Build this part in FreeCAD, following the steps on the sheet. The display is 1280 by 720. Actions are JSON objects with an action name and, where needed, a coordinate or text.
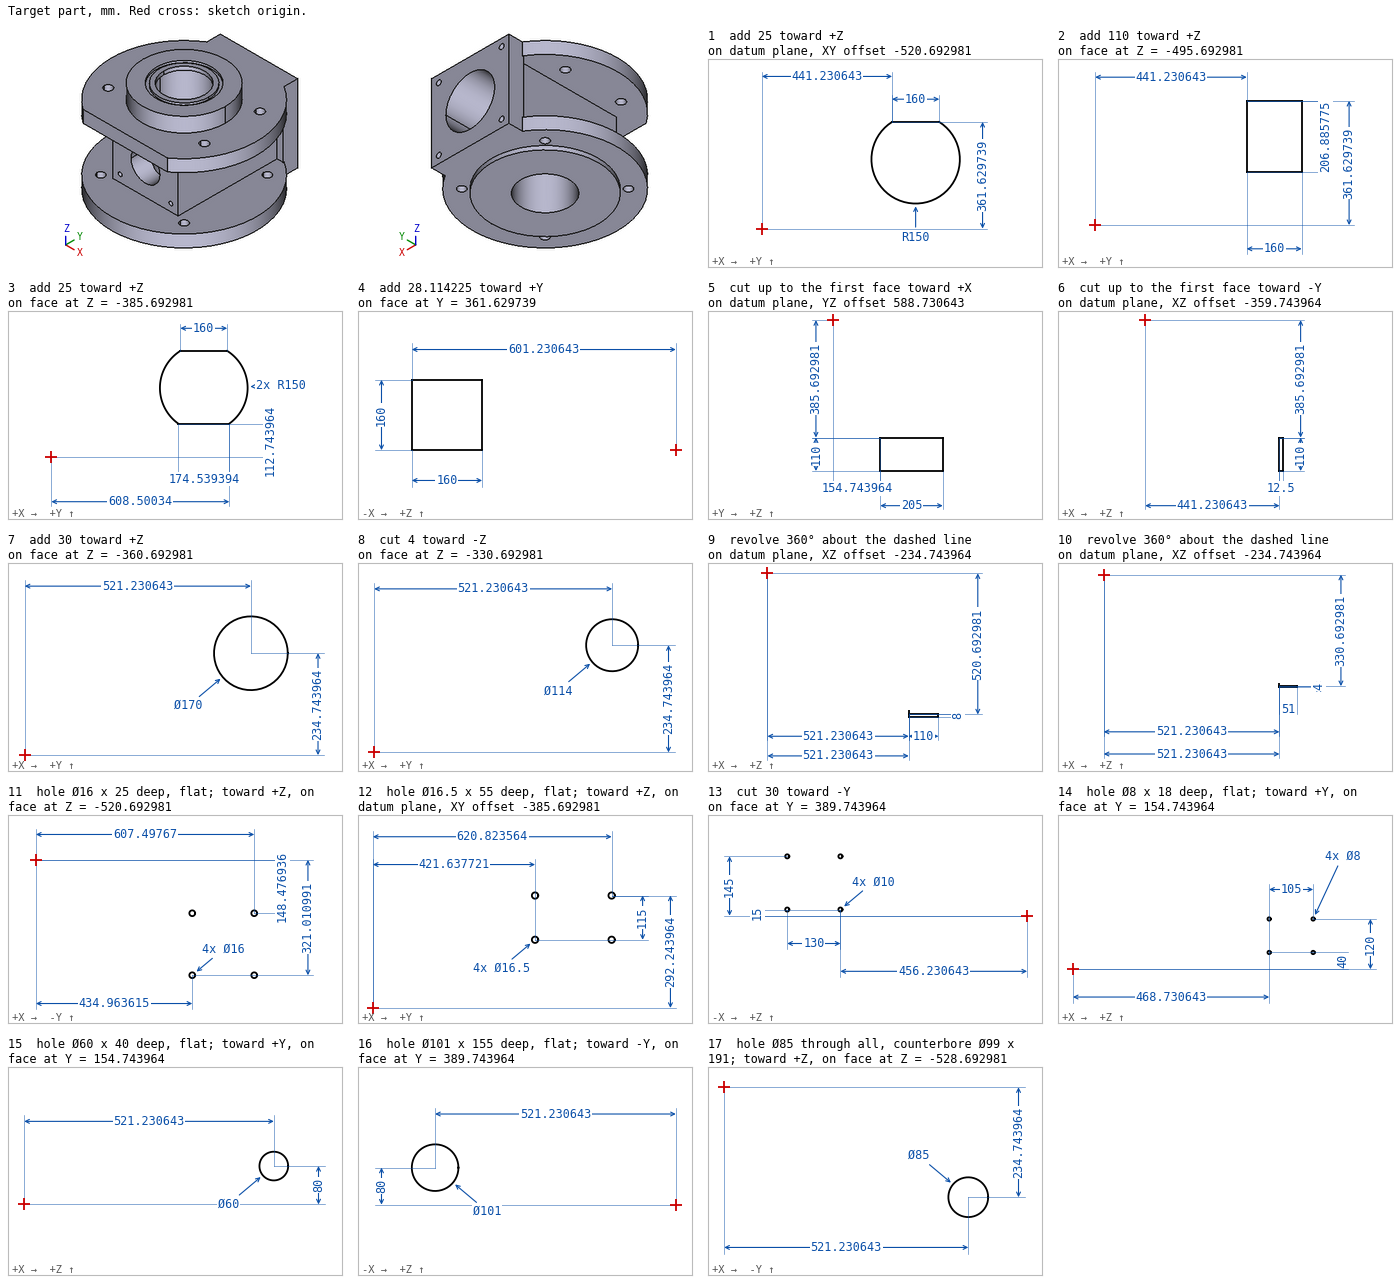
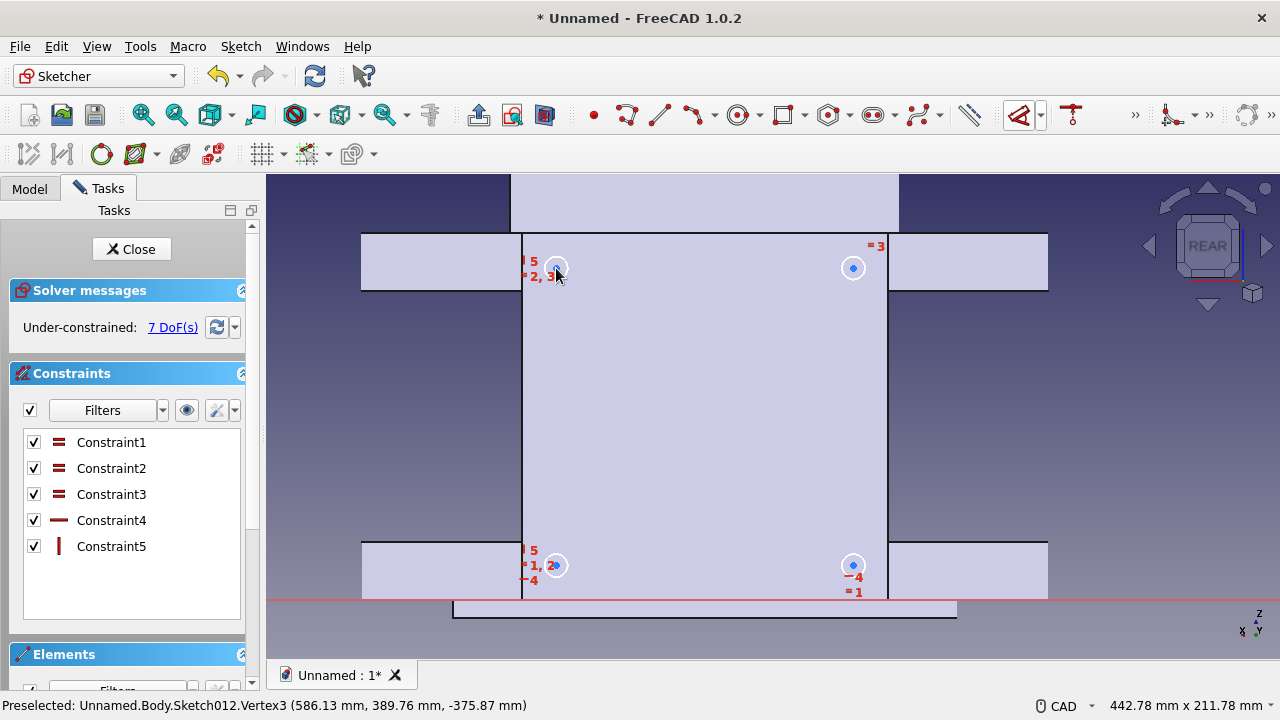
{"action": "left_click", "coordinate": [854, 566]}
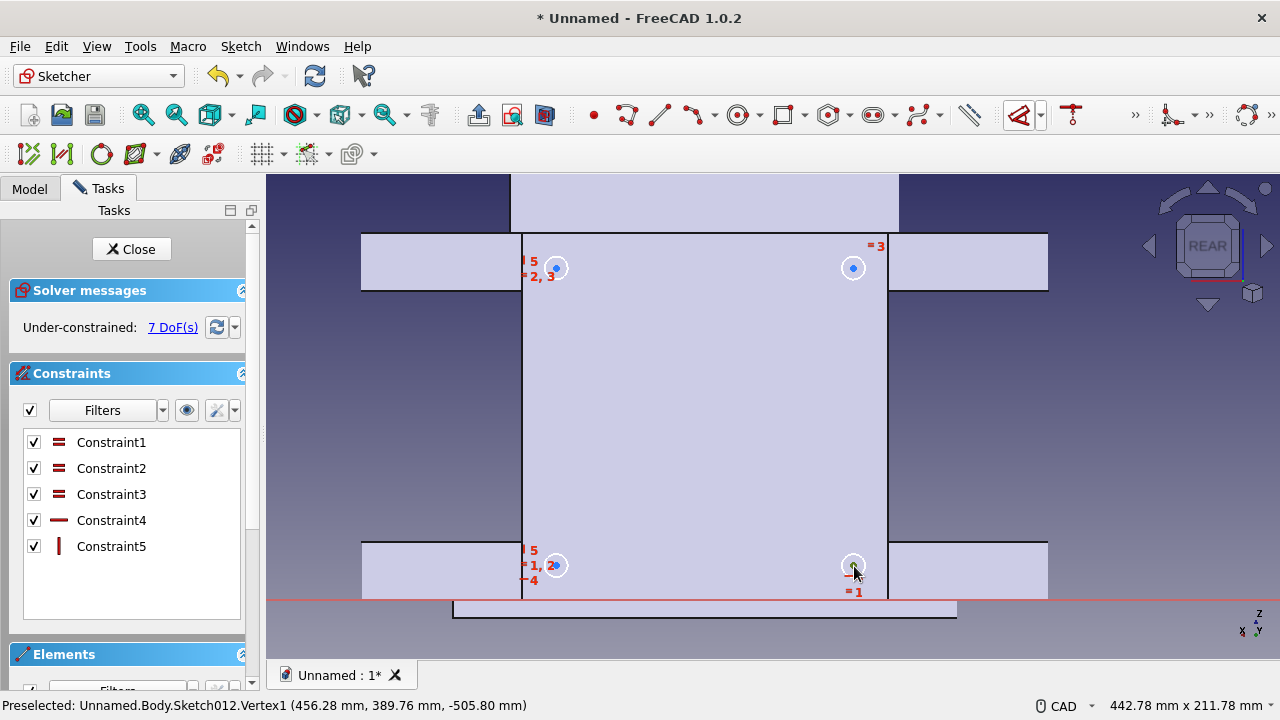
{"action": "left_click", "coordinate": [853, 268]}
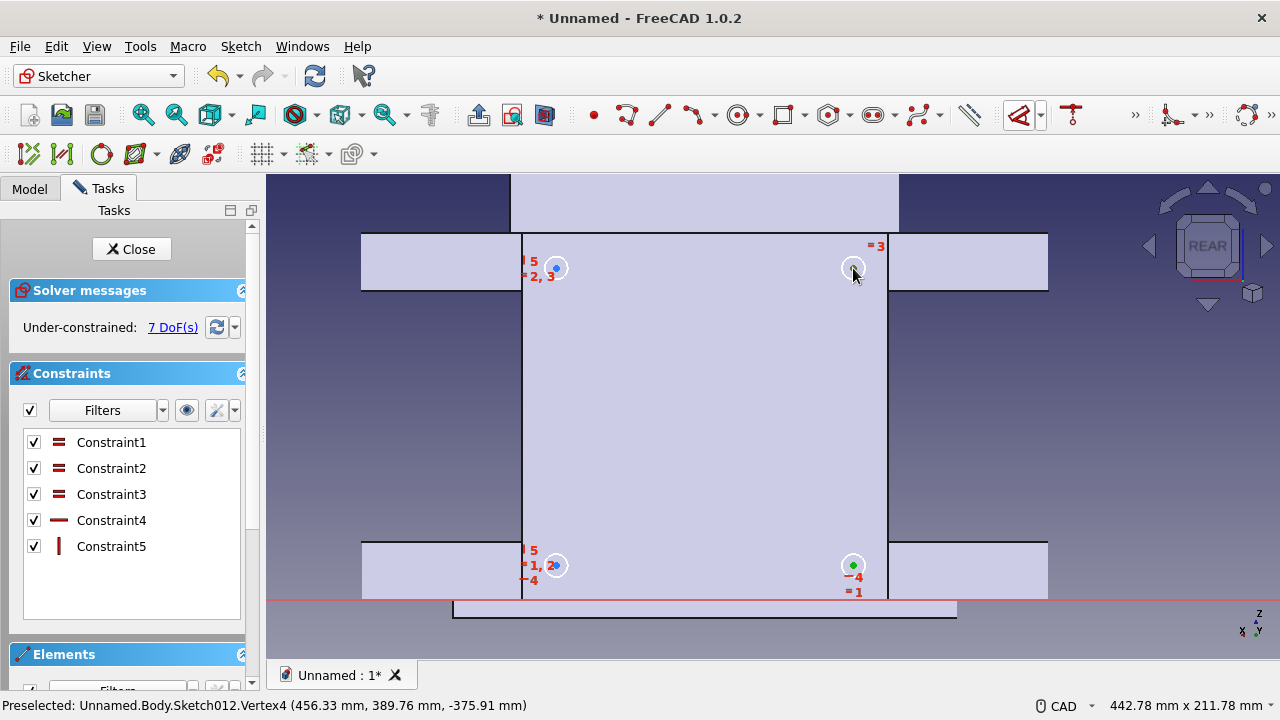
{"action": "key", "text": "v"}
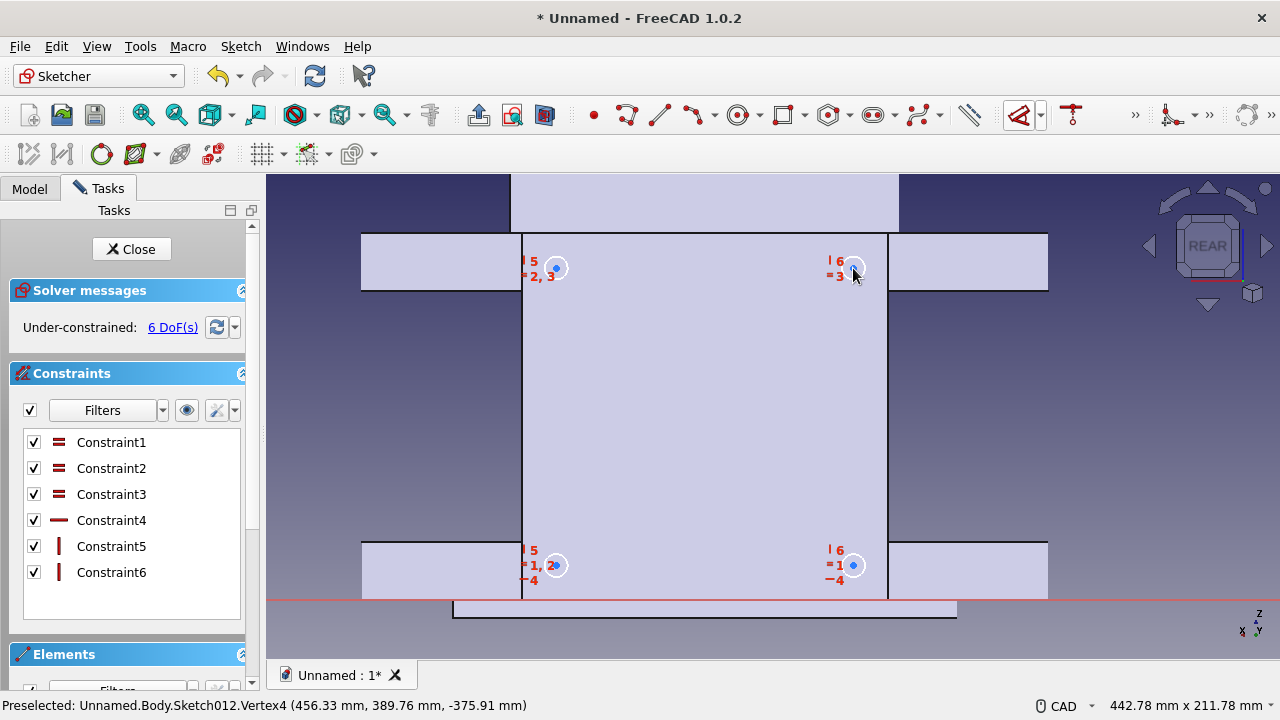
{"action": "left_click", "coordinate": [556, 268]}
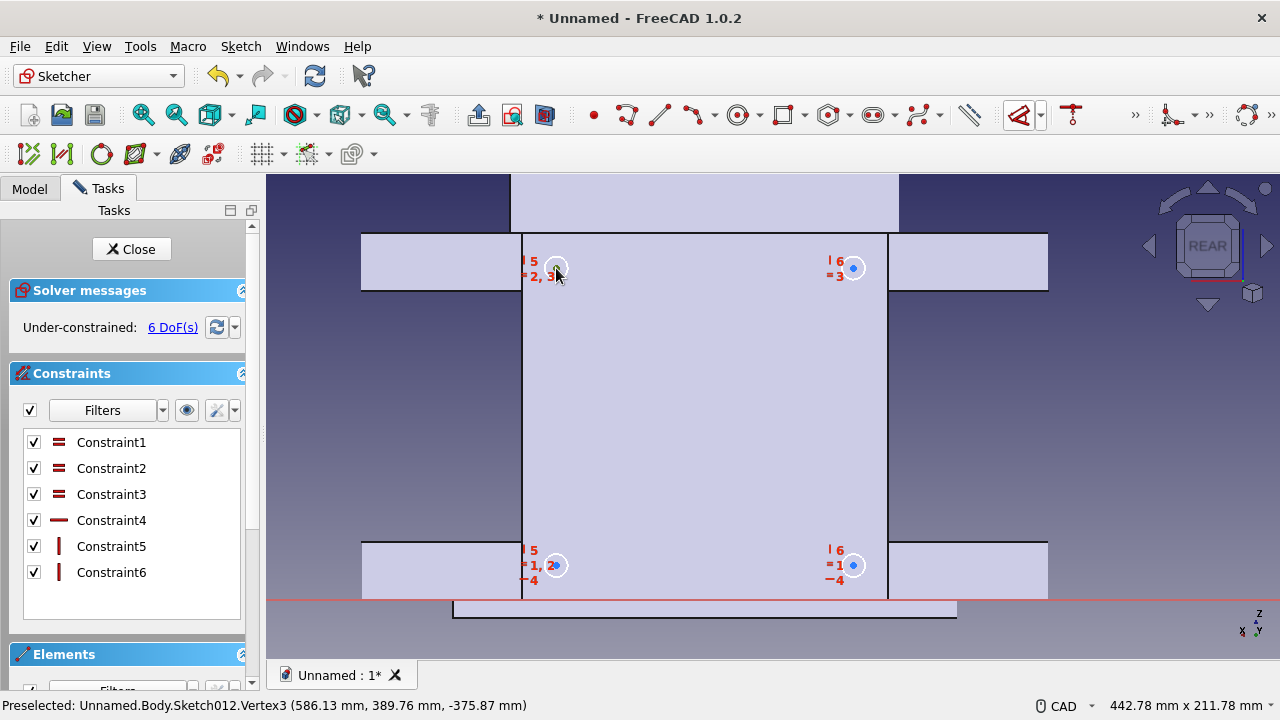
{"action": "left_click", "coordinate": [854, 268]}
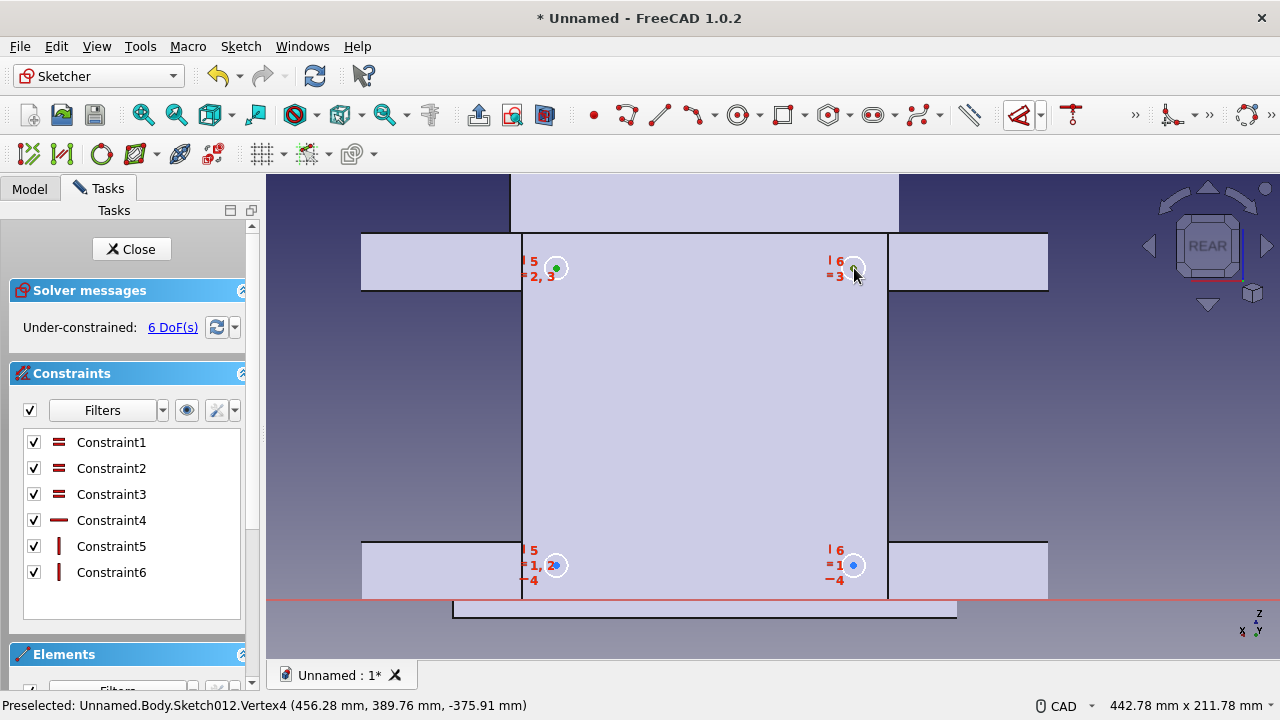
{"action": "key", "text": "h"}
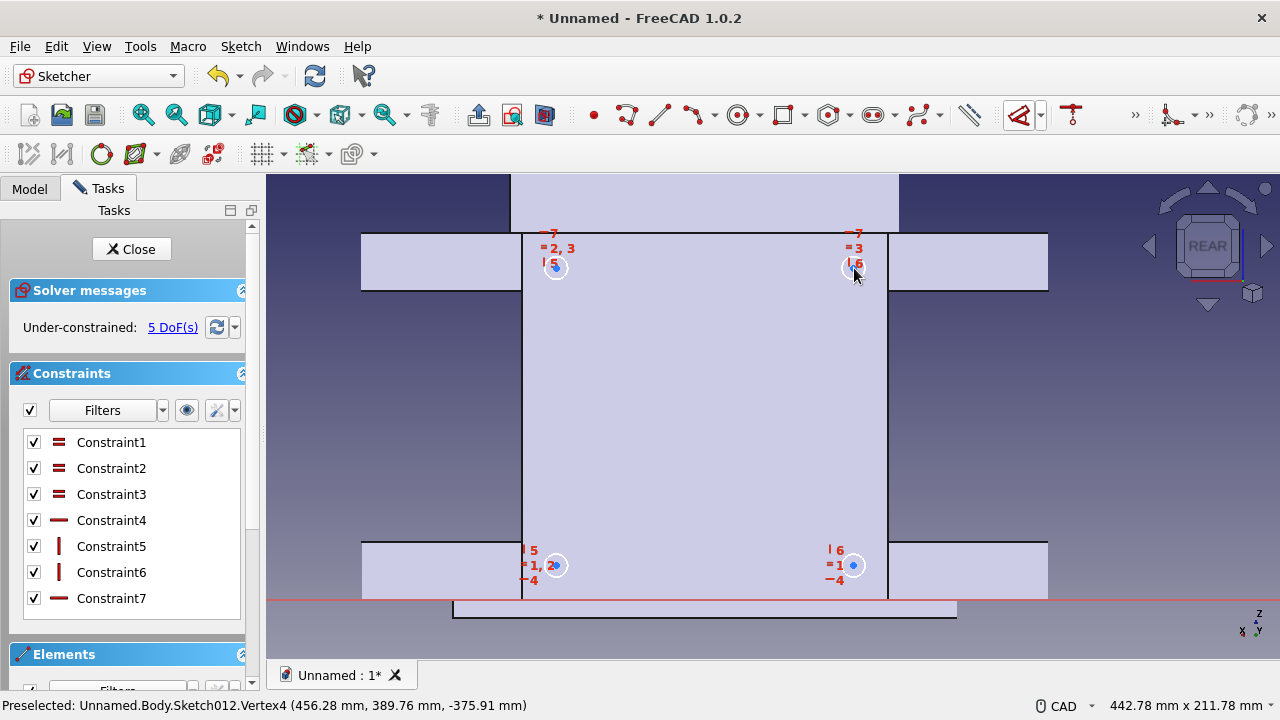
{"action": "scroll", "coordinate": [862, 557], "scroll_direction": "up", "scroll_amount": 3}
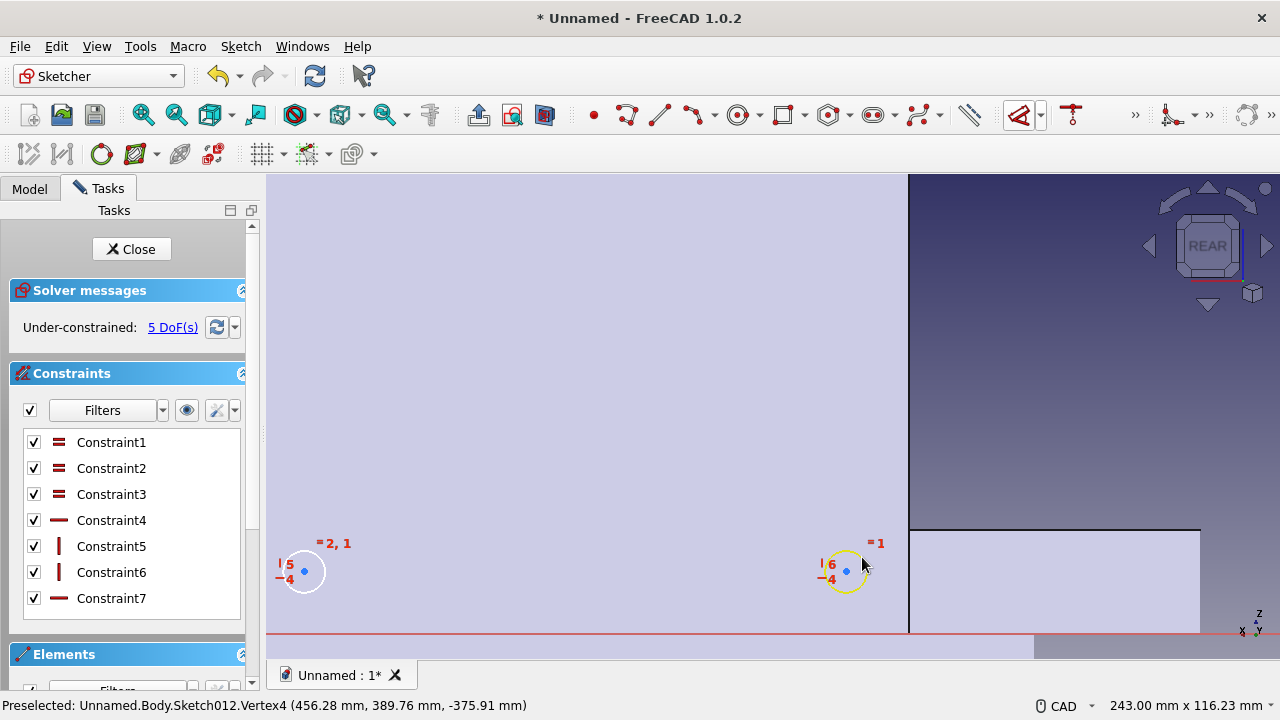
{"action": "left_click", "coordinate": [861, 557]}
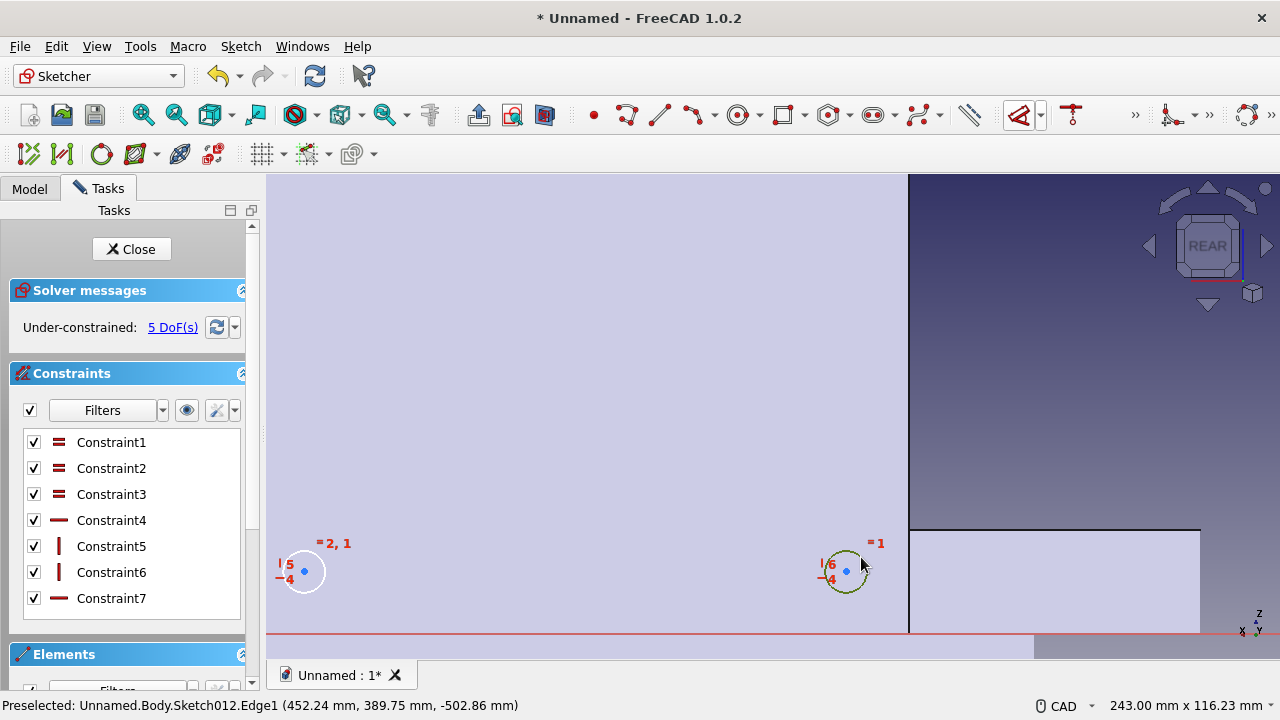
{"action": "left_click", "coordinate": [1040, 116]}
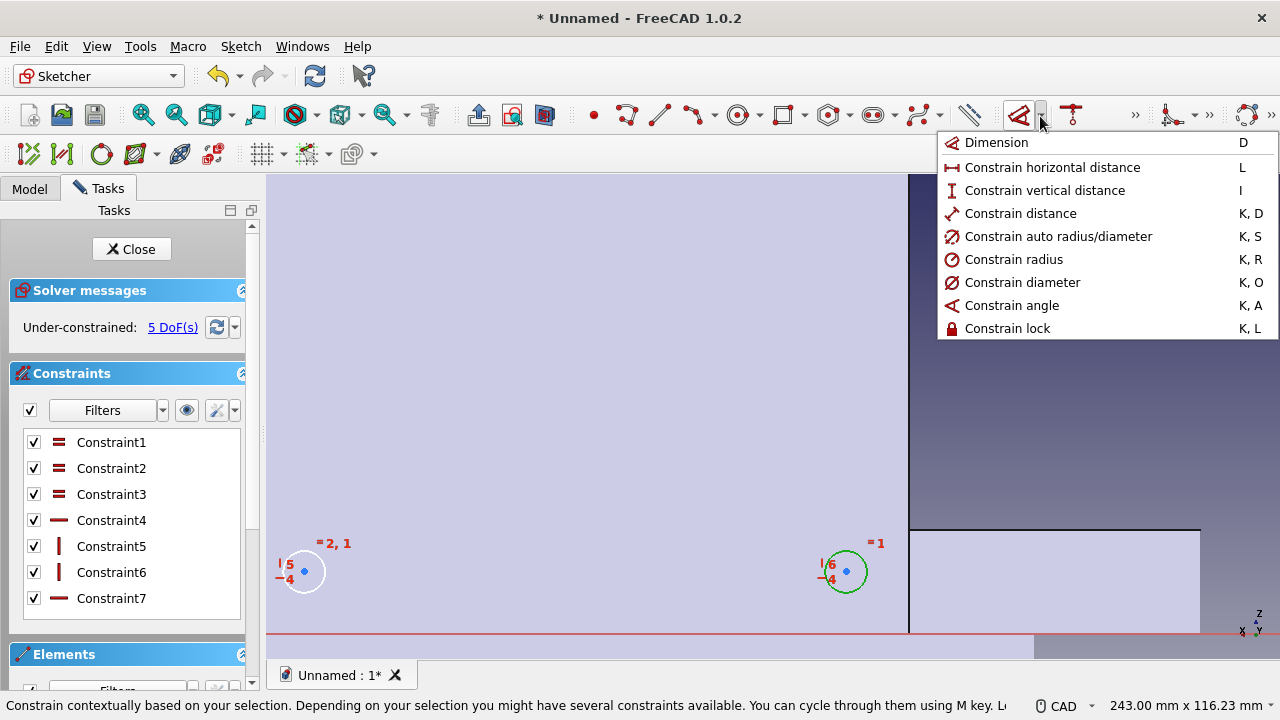
{"action": "left_click", "coordinate": [1108, 282]}